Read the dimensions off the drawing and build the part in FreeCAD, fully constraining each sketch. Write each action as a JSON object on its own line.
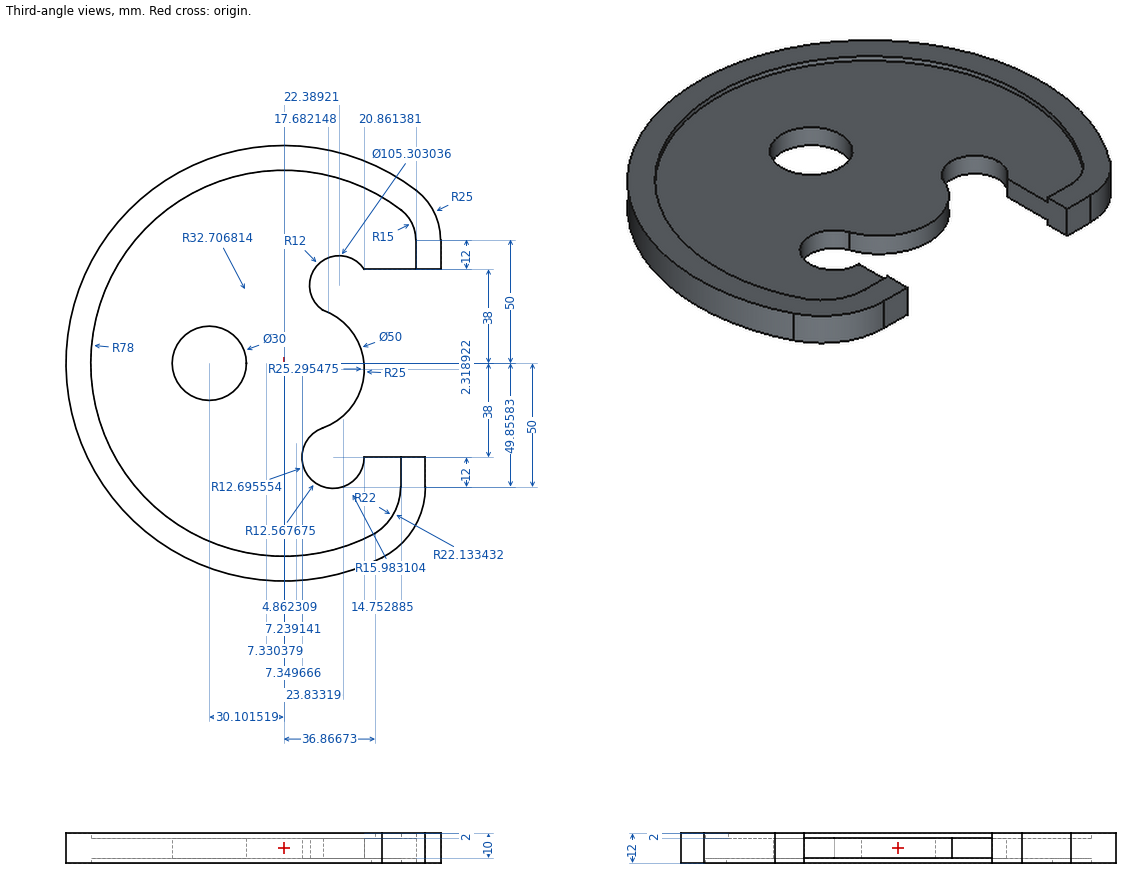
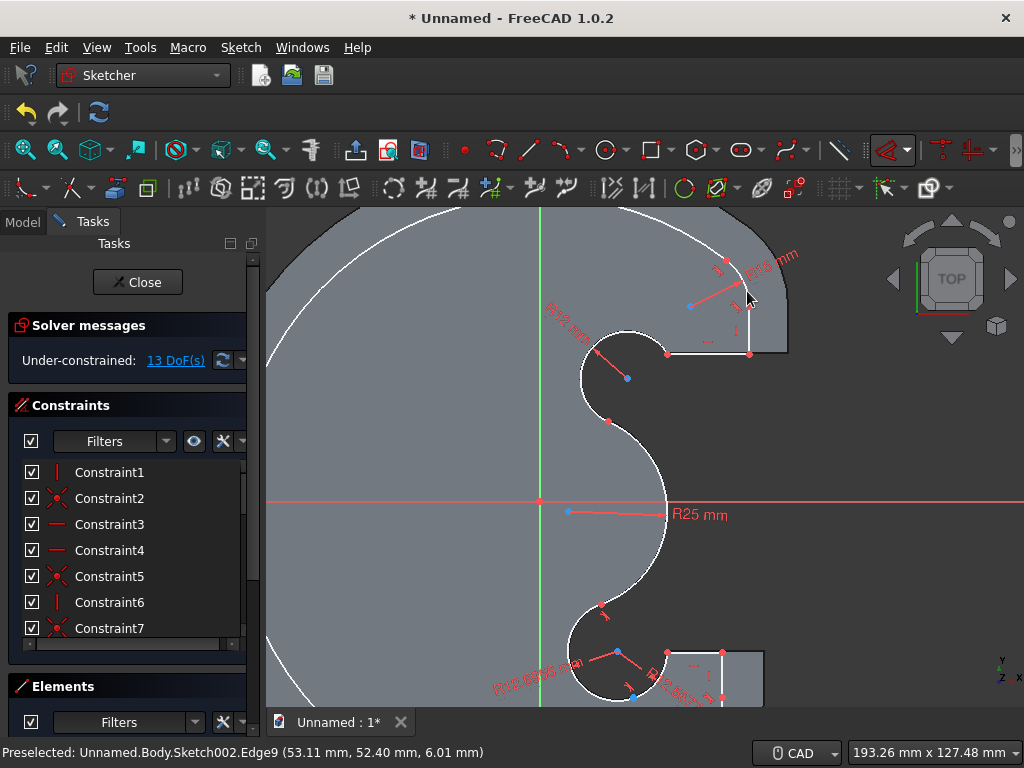
{"action": "left_click", "coordinate": [360, 255]}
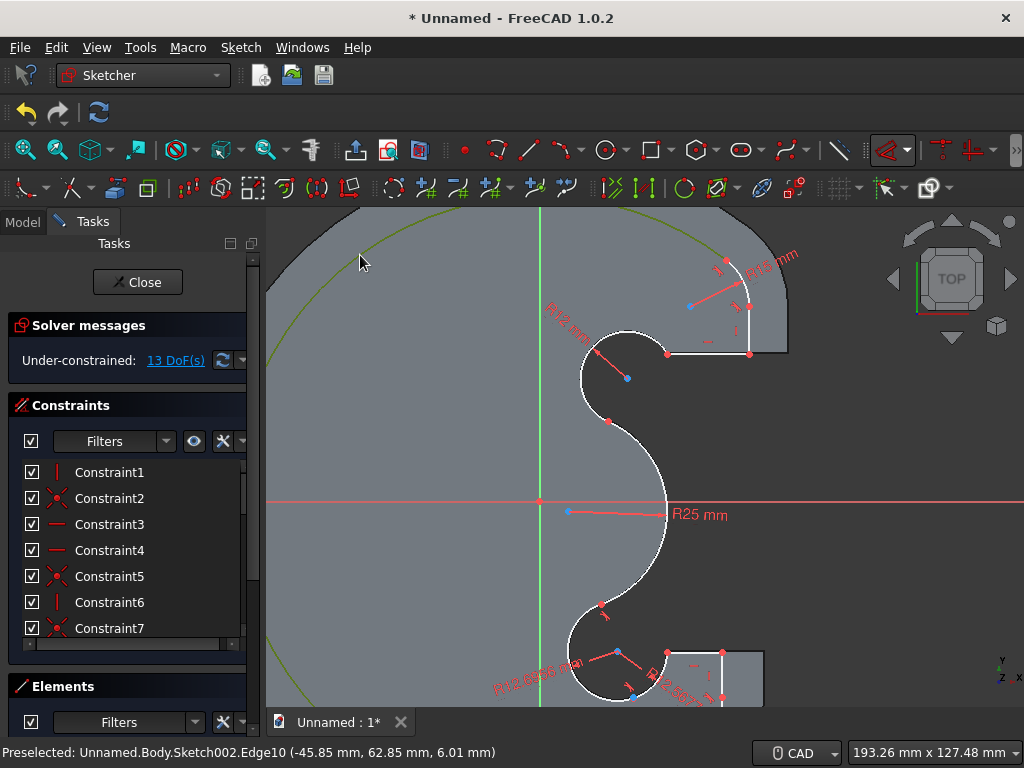
{"action": "key", "text": "k r"}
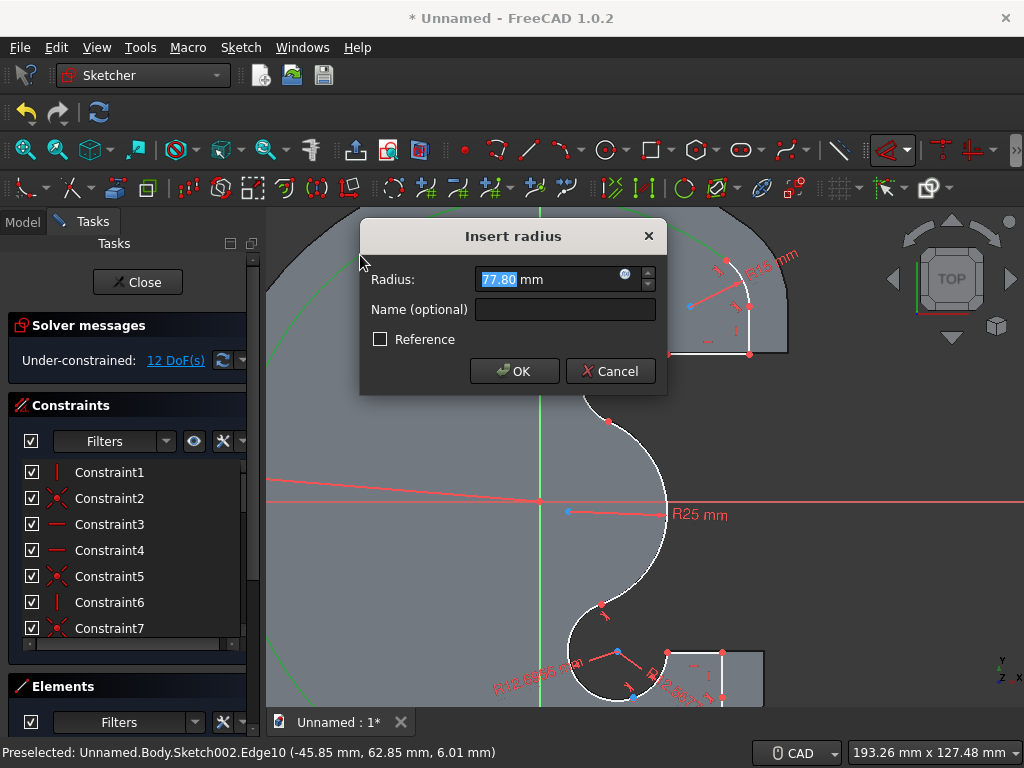
{"action": "type", "text": "78"}
{"action": "key", "text": "Return"}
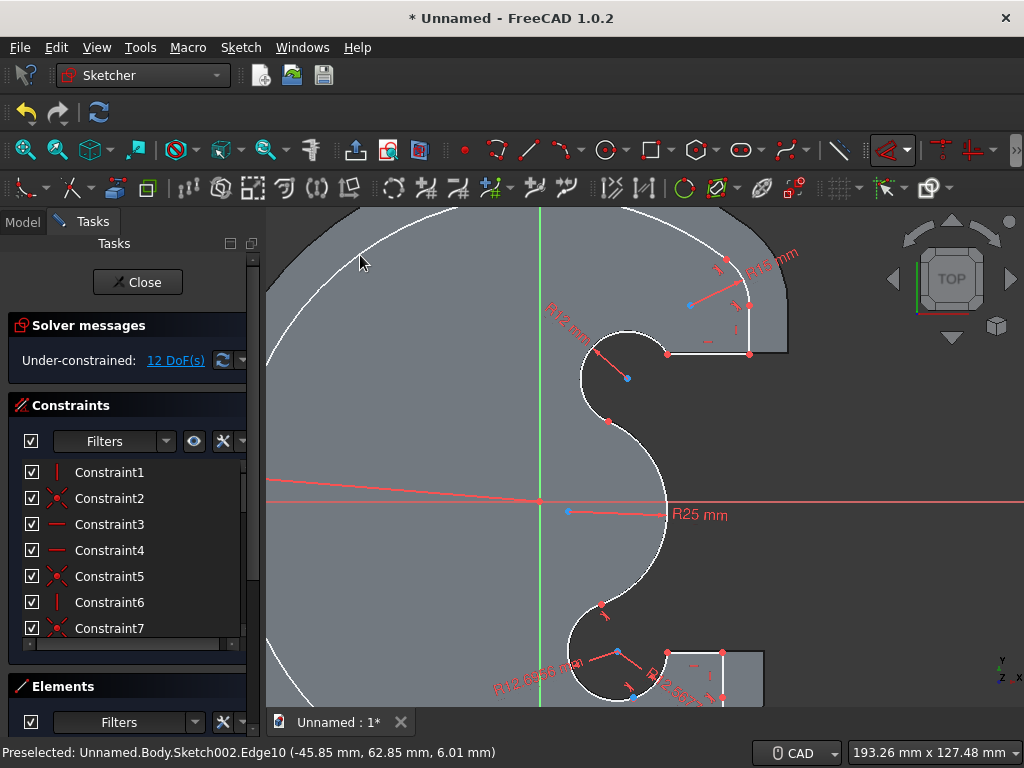
{"action": "scroll", "coordinate": [749, 339], "scroll_direction": "down", "scroll_amount": 2}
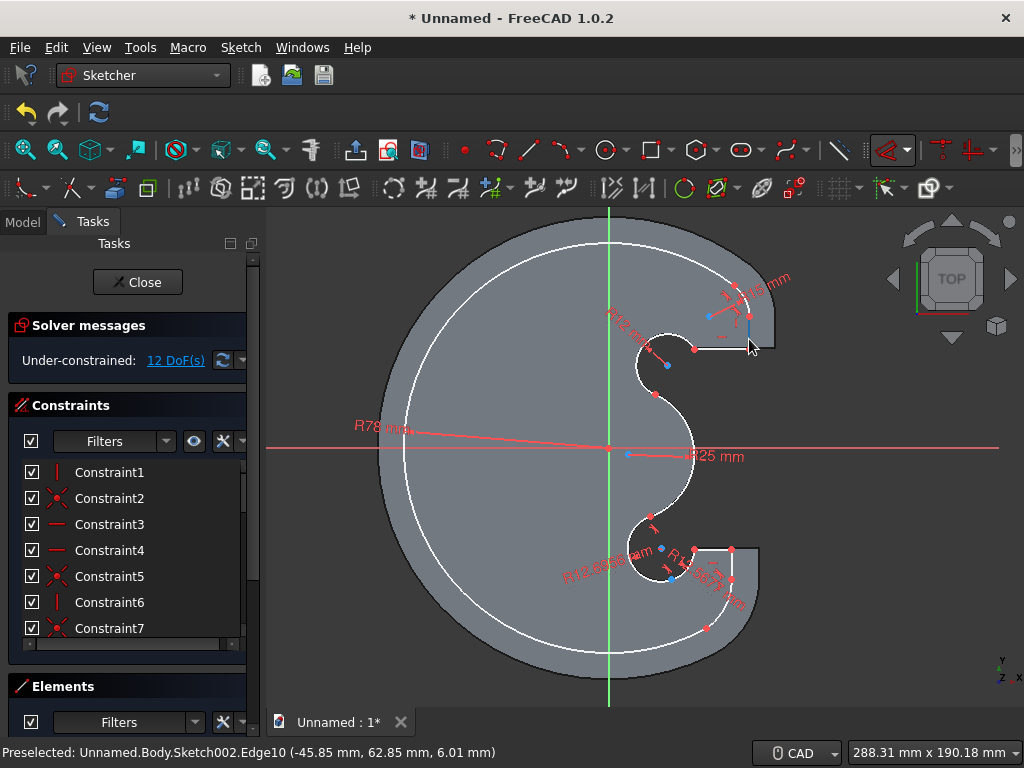
{"action": "left_click", "coordinate": [719, 617]}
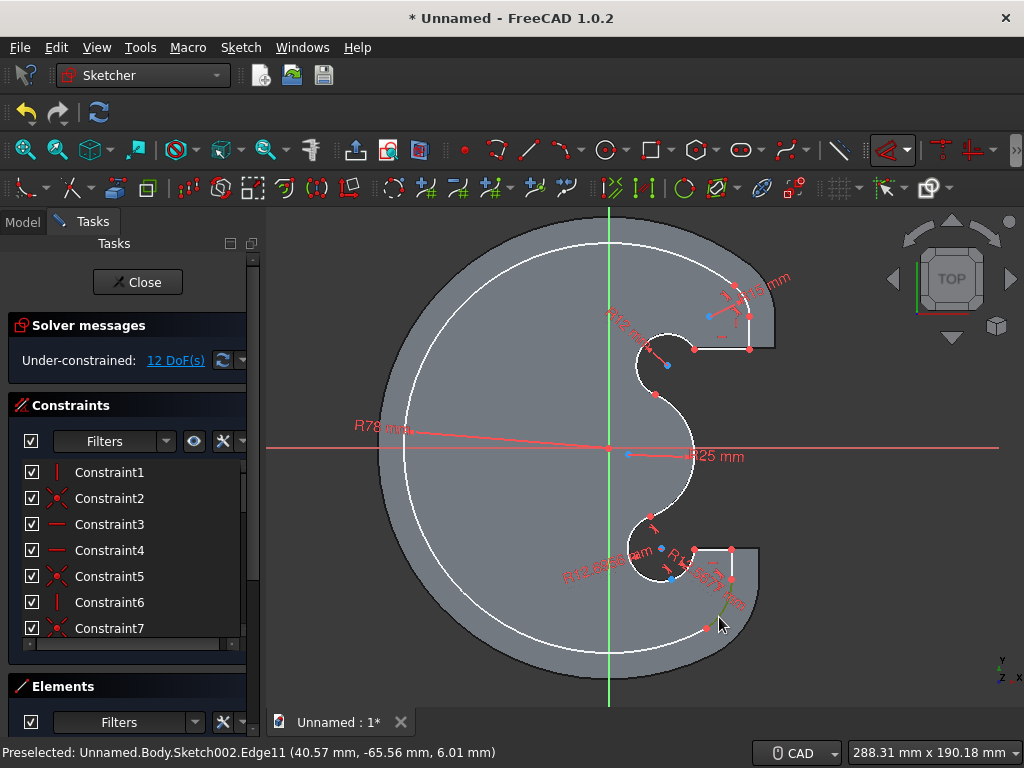
{"action": "key", "text": "k r"}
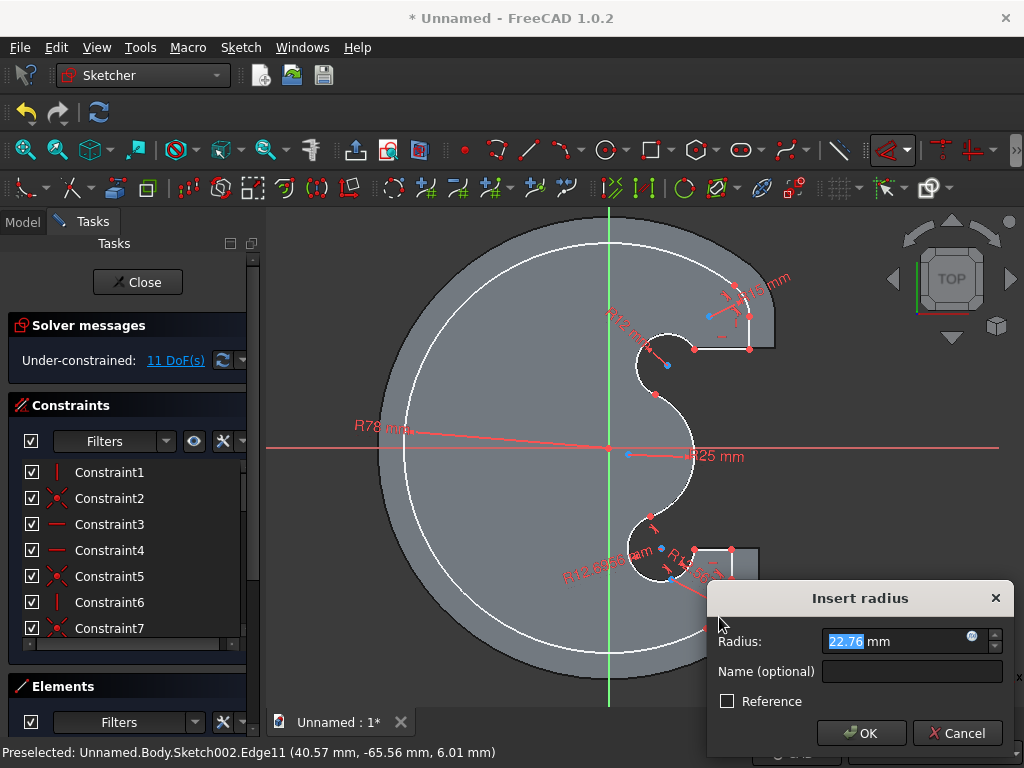
{"action": "type", "text": "22.133432"}
{"action": "key", "text": "Return"}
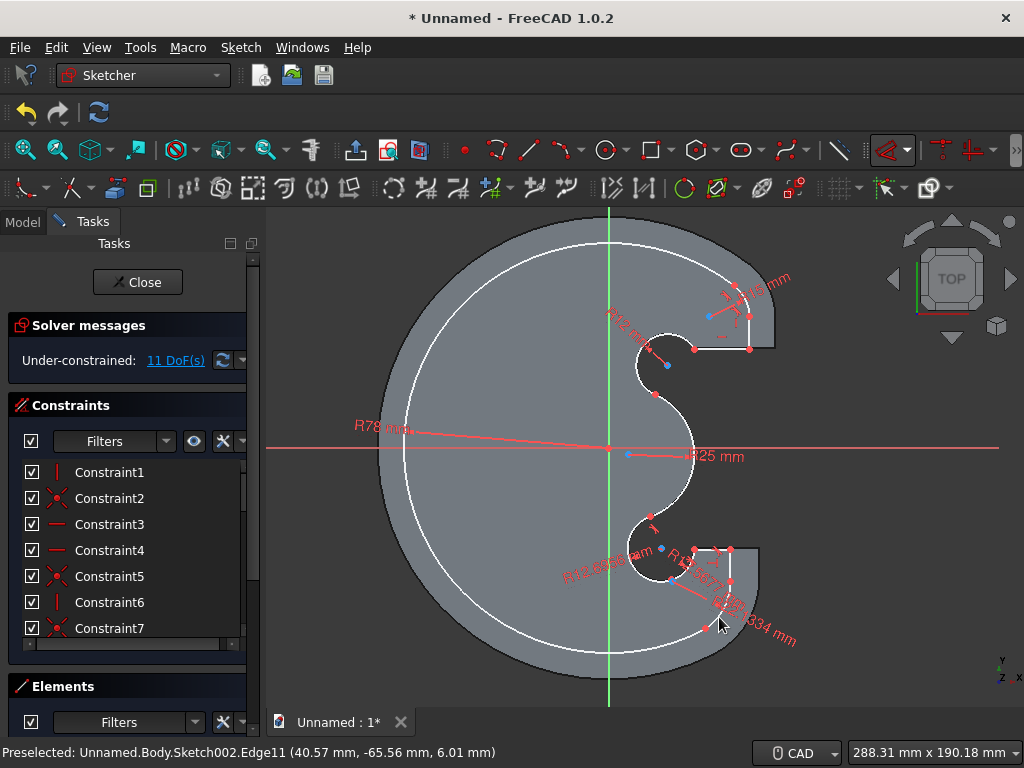
{"action": "scroll", "coordinate": [730, 572], "scroll_direction": "up", "scroll_amount": 2}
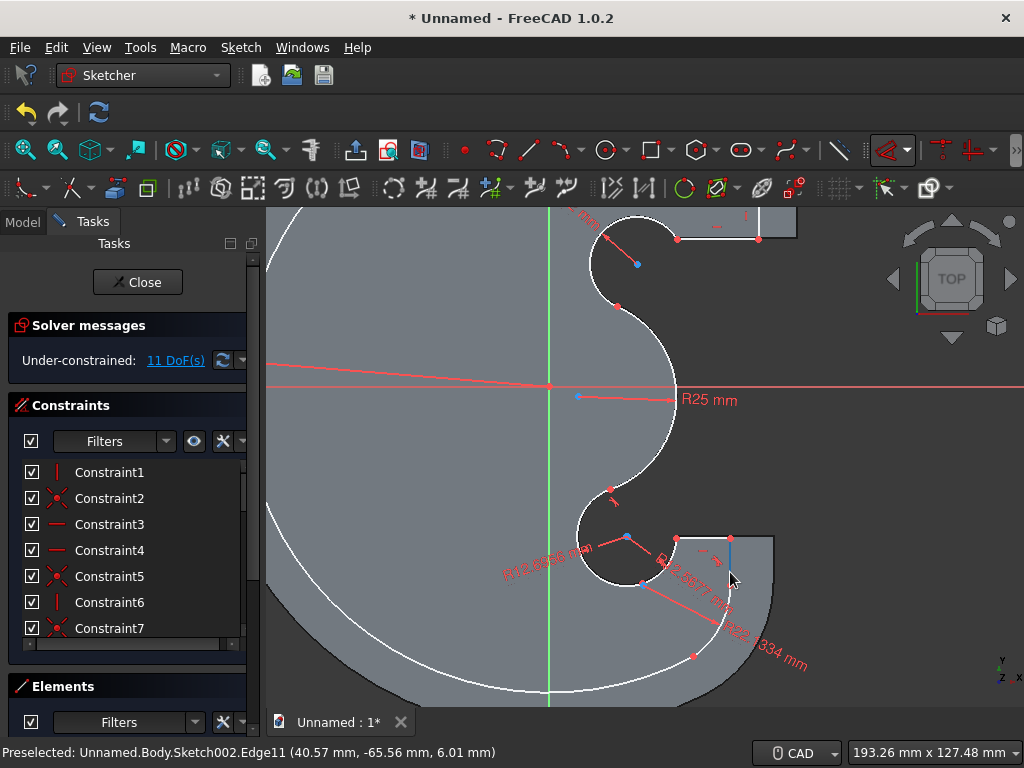
{"action": "left_click", "coordinate": [730, 571]}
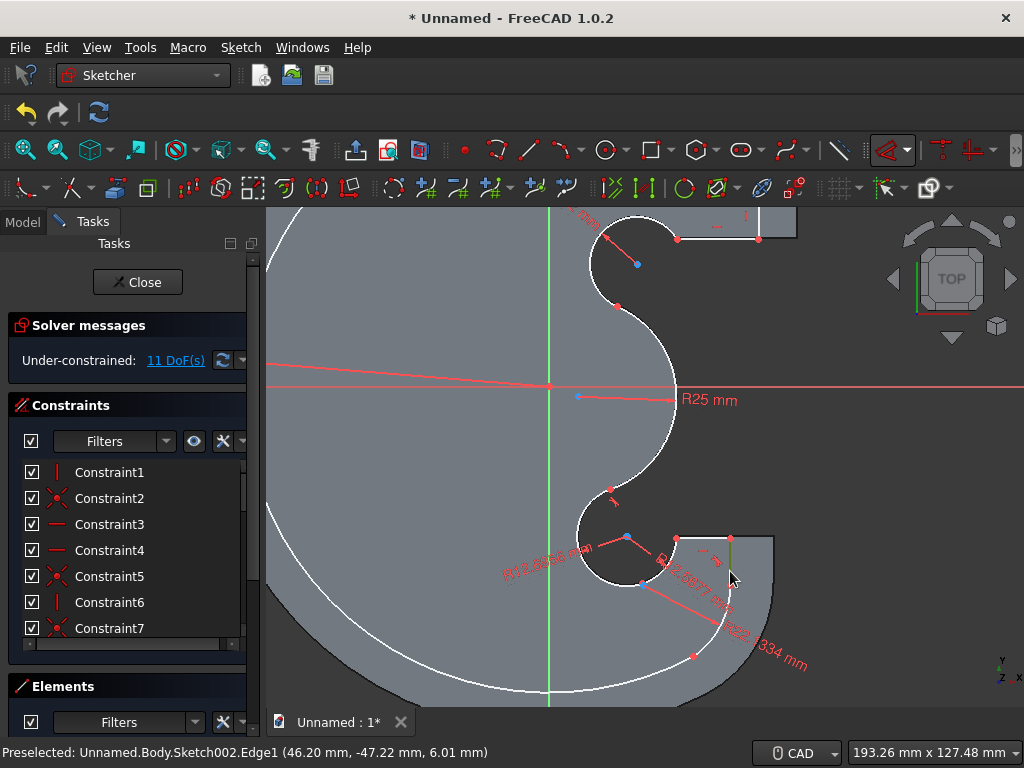
{"action": "key", "text": "i"}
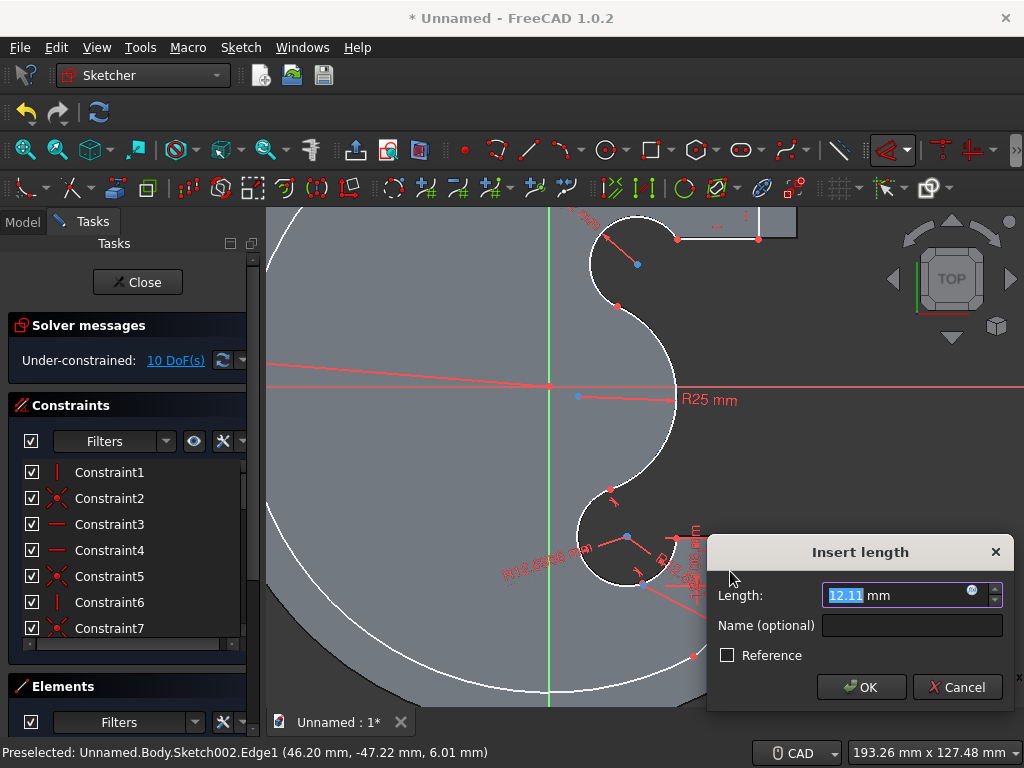
{"action": "type", "text": "12"}
{"action": "key", "text": "Return"}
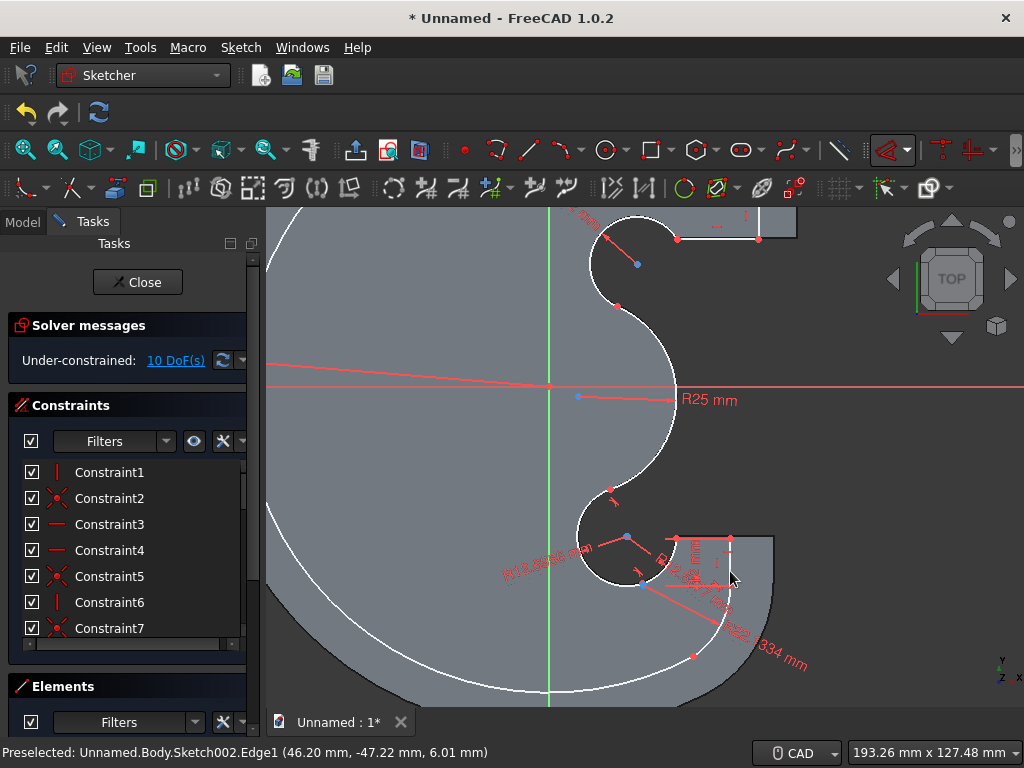
{"action": "scroll", "coordinate": [730, 573], "scroll_direction": "down", "scroll_amount": 2}